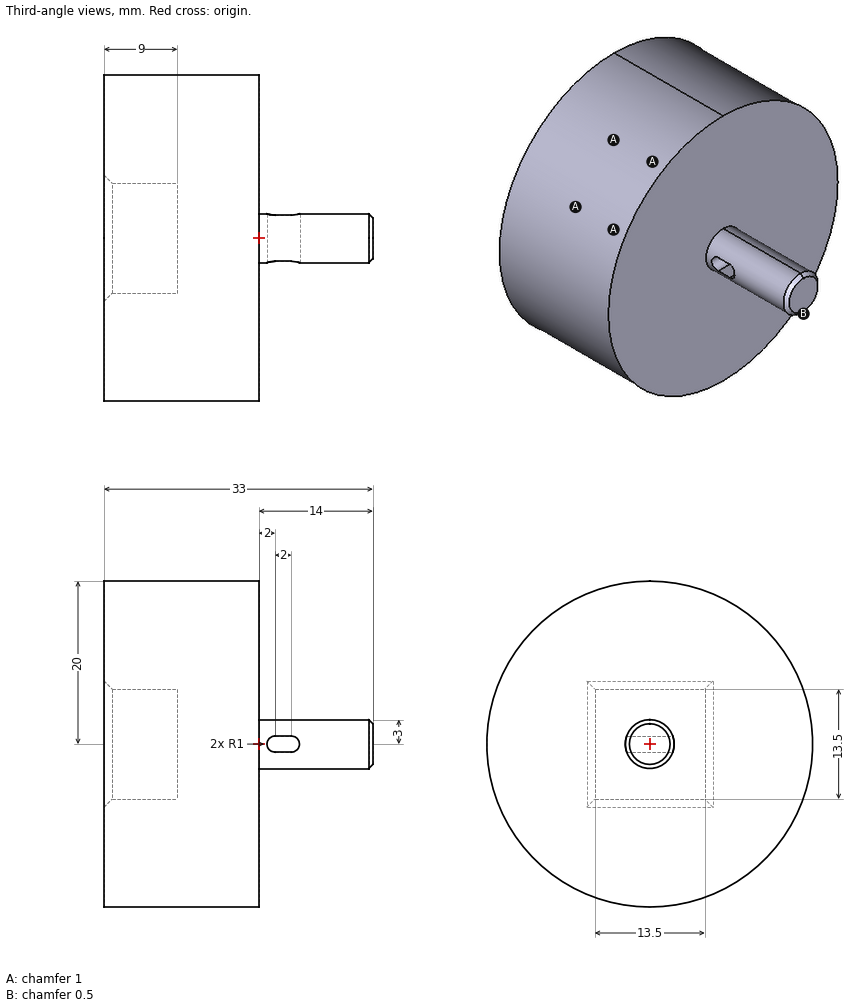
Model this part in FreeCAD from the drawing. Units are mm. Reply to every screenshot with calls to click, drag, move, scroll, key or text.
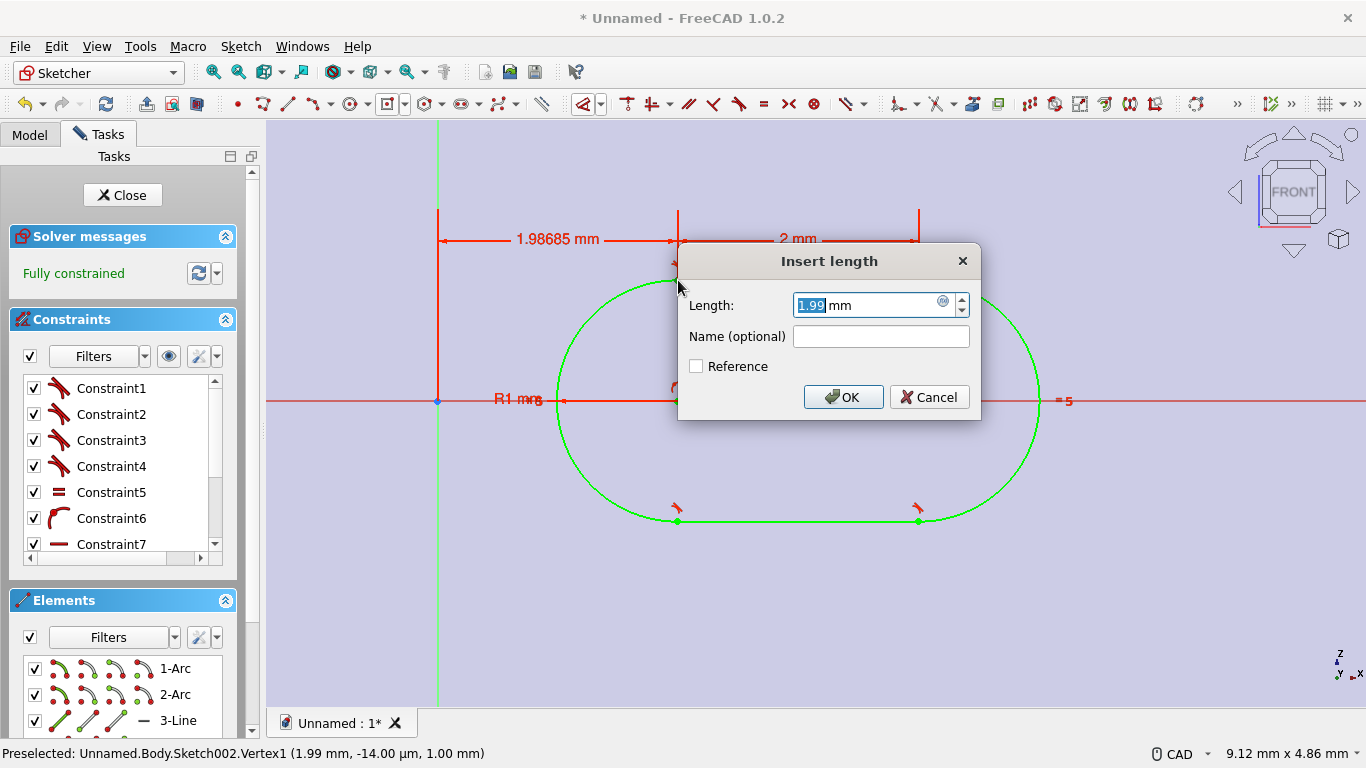
text(2)
key(Return)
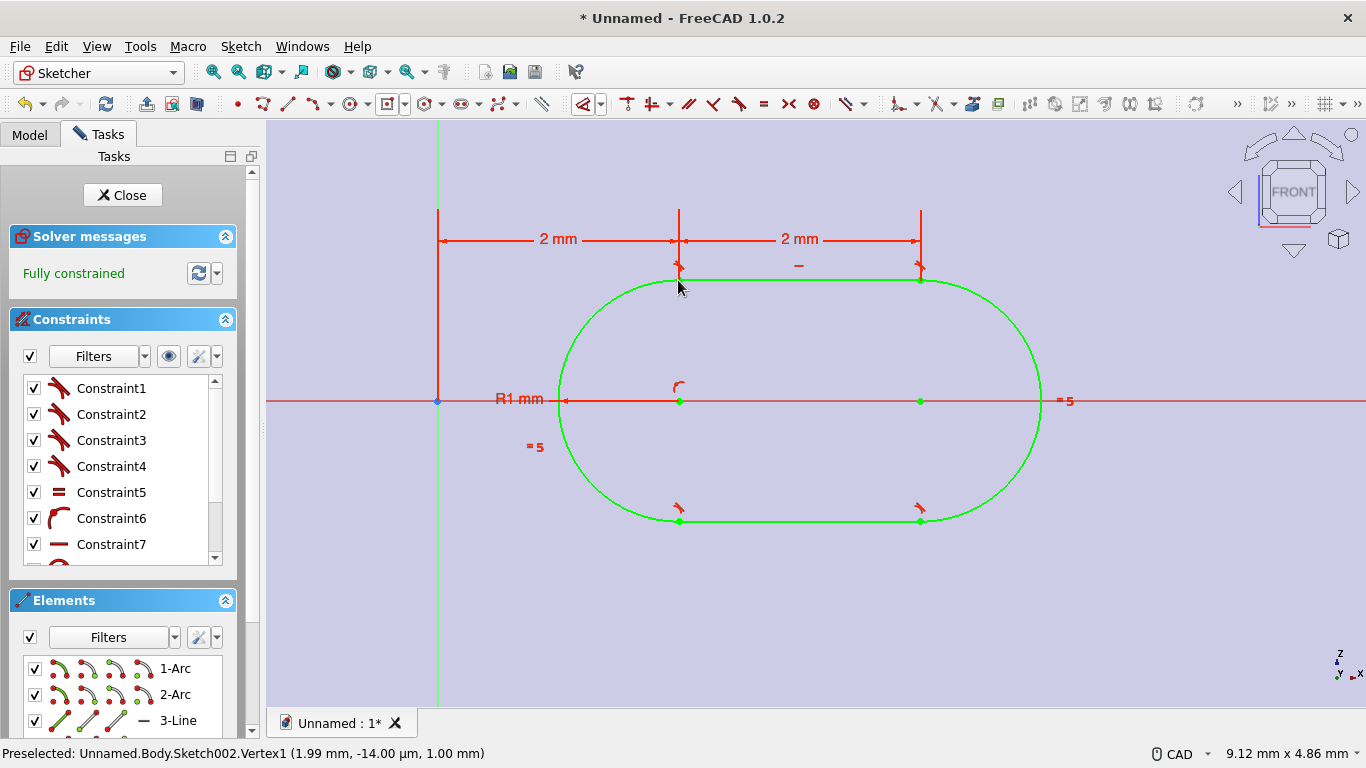
click(123, 195)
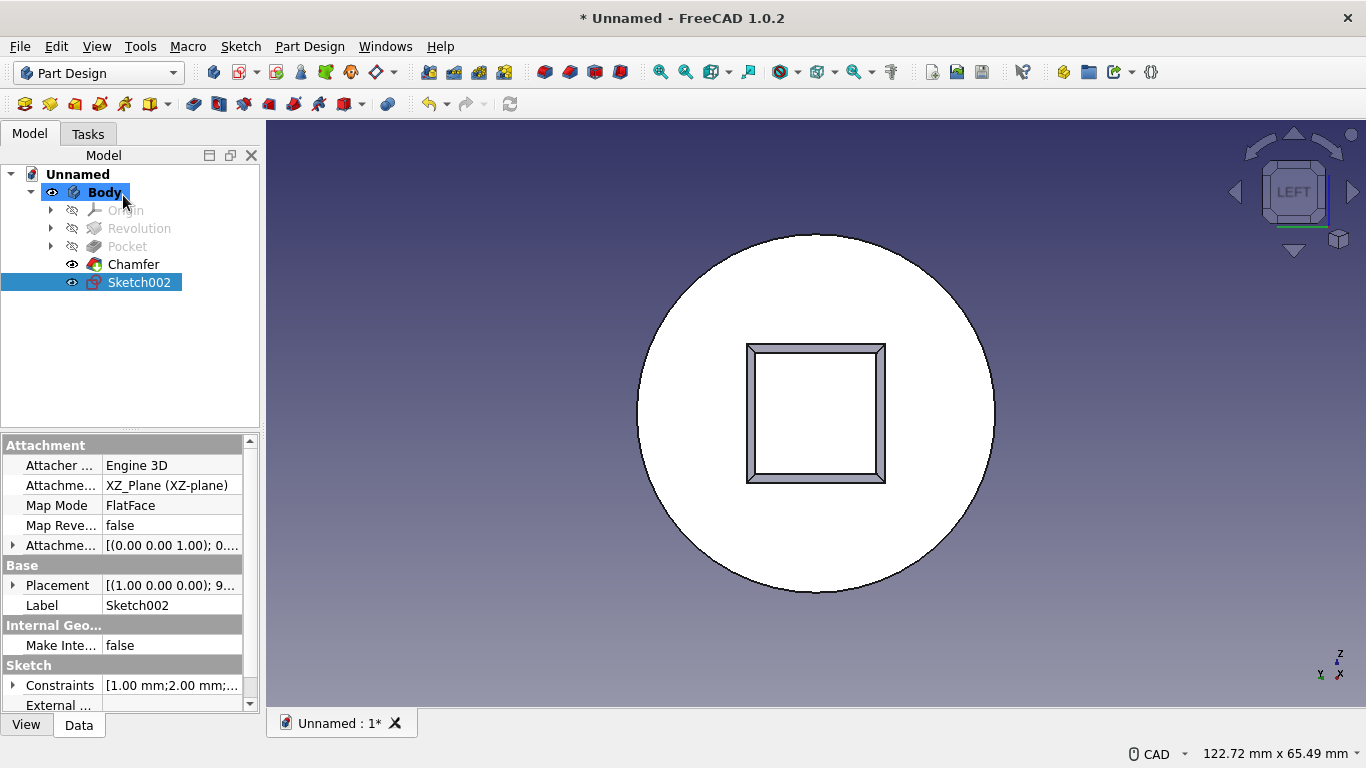
click(194, 104)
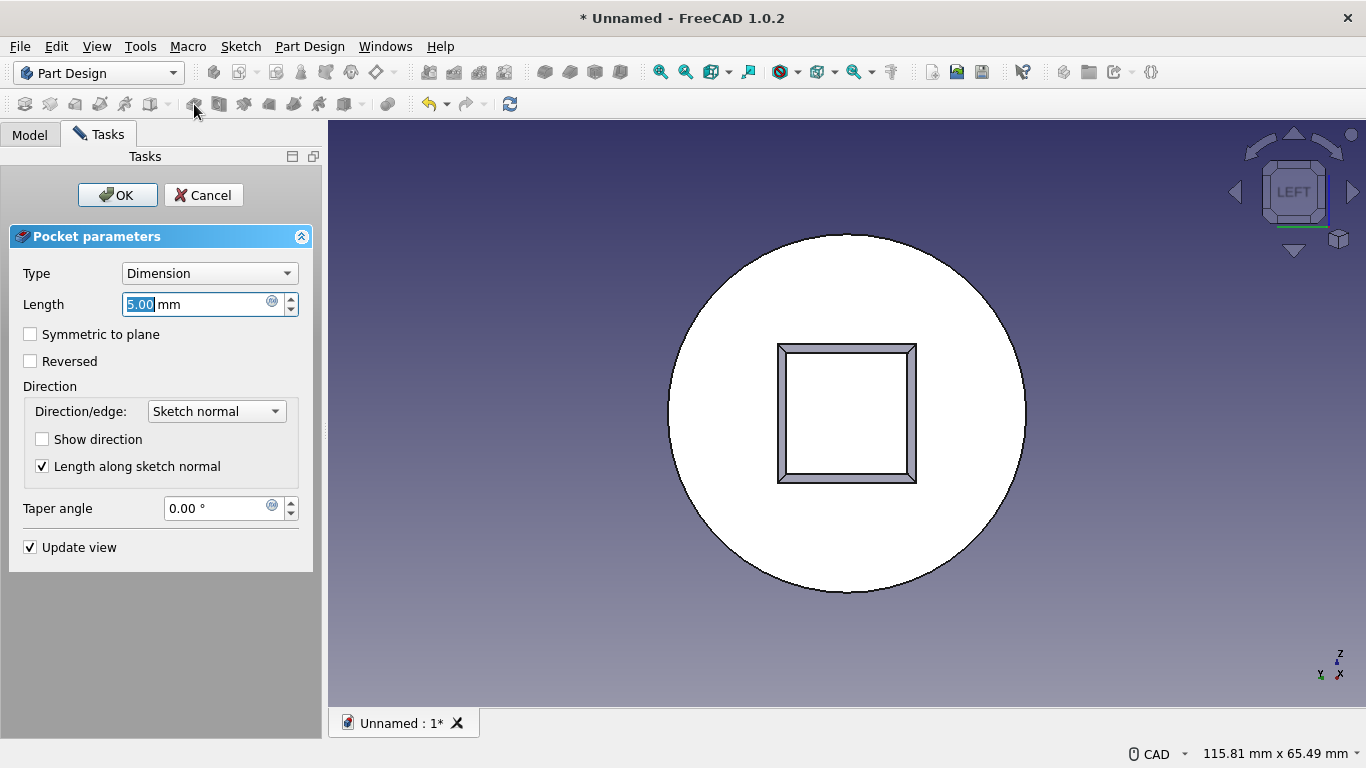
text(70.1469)
key(Tab)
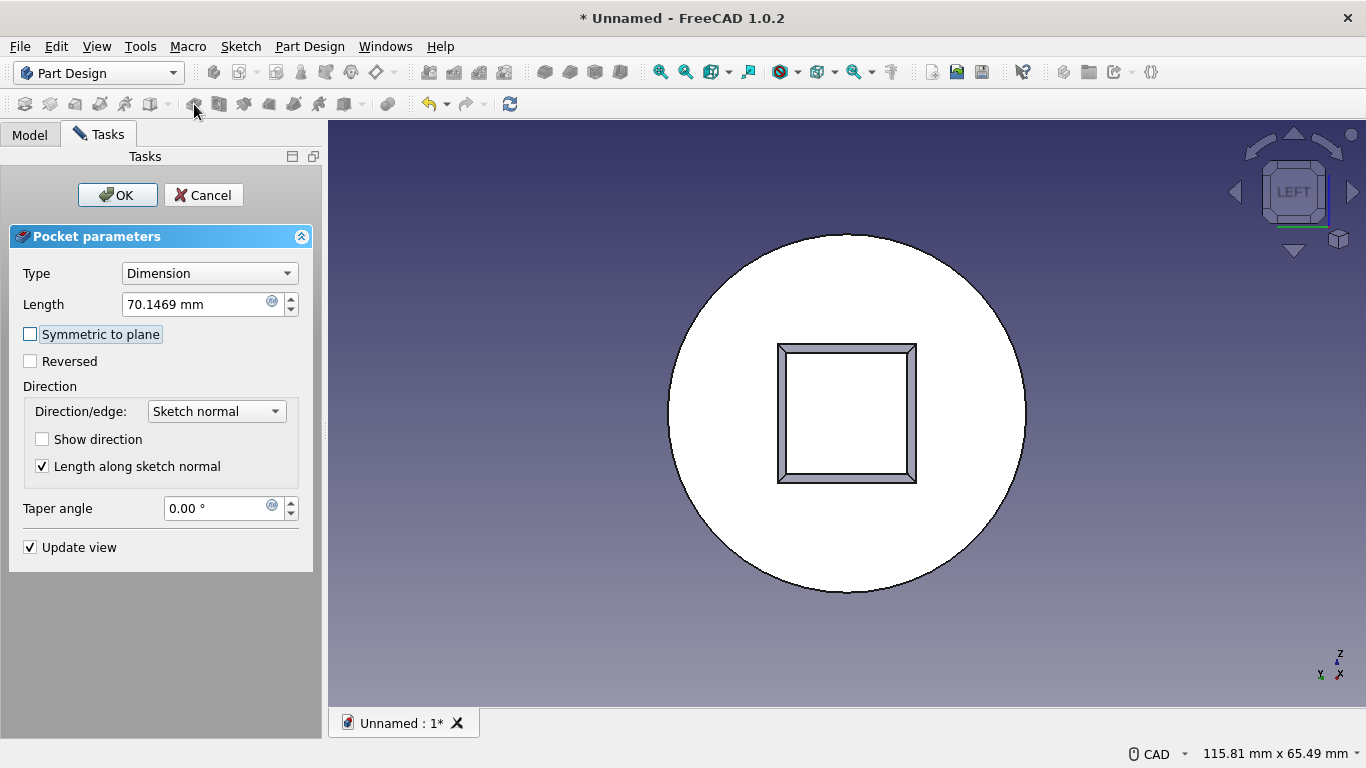
click(31, 334)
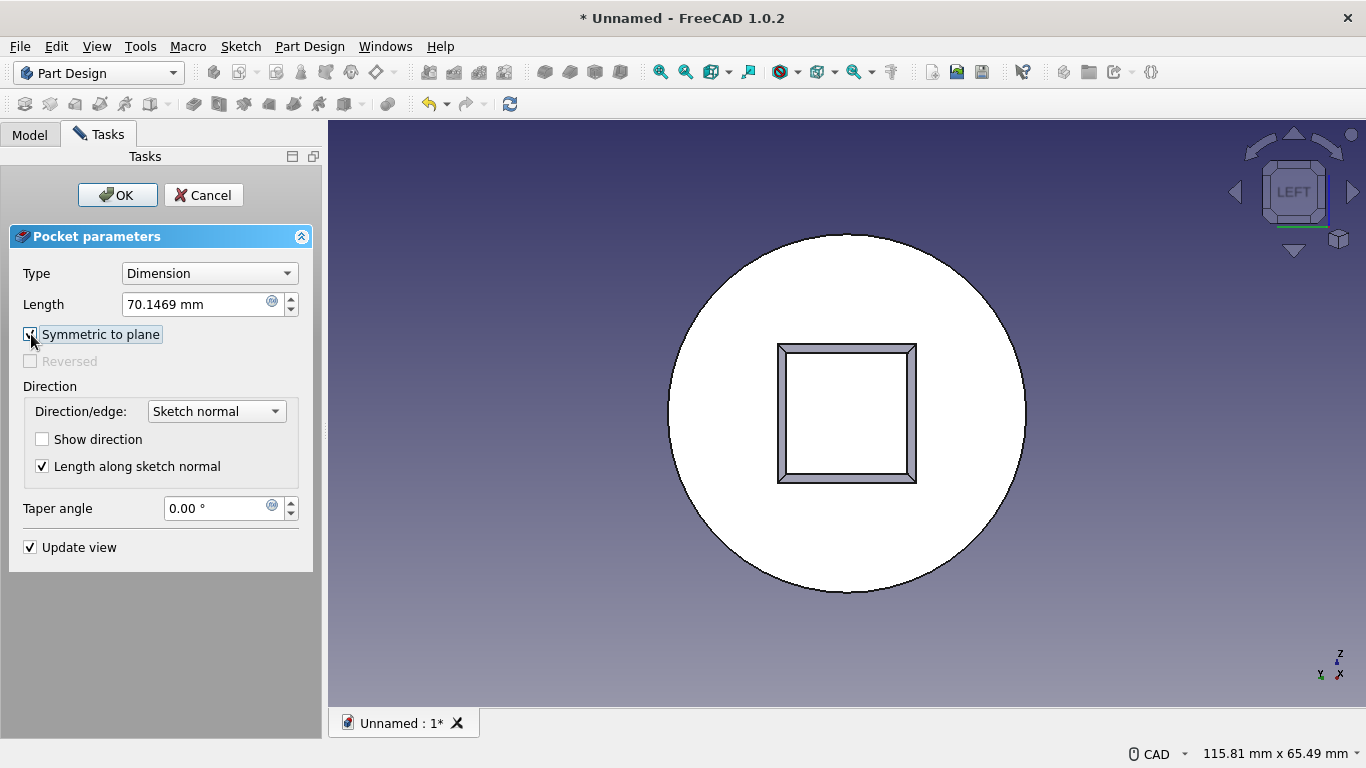
click(118, 195)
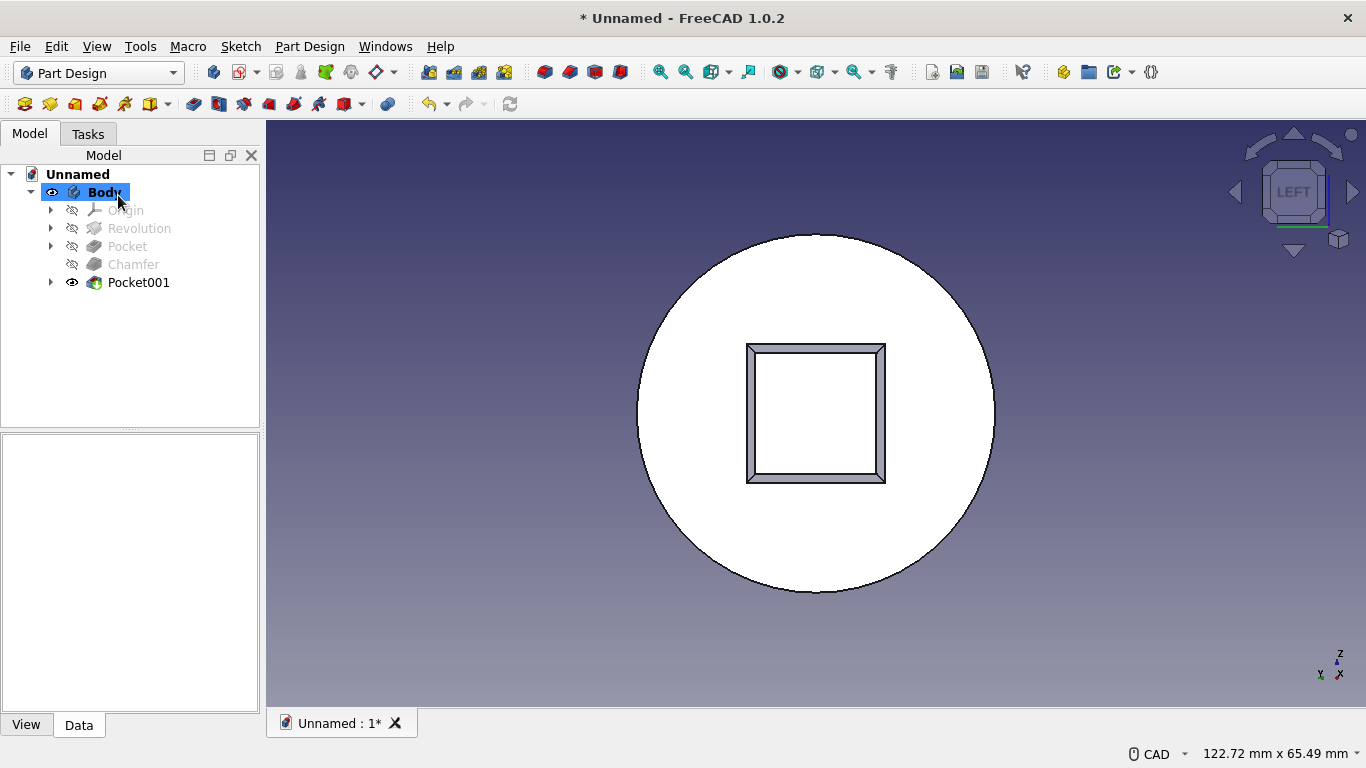
key(0)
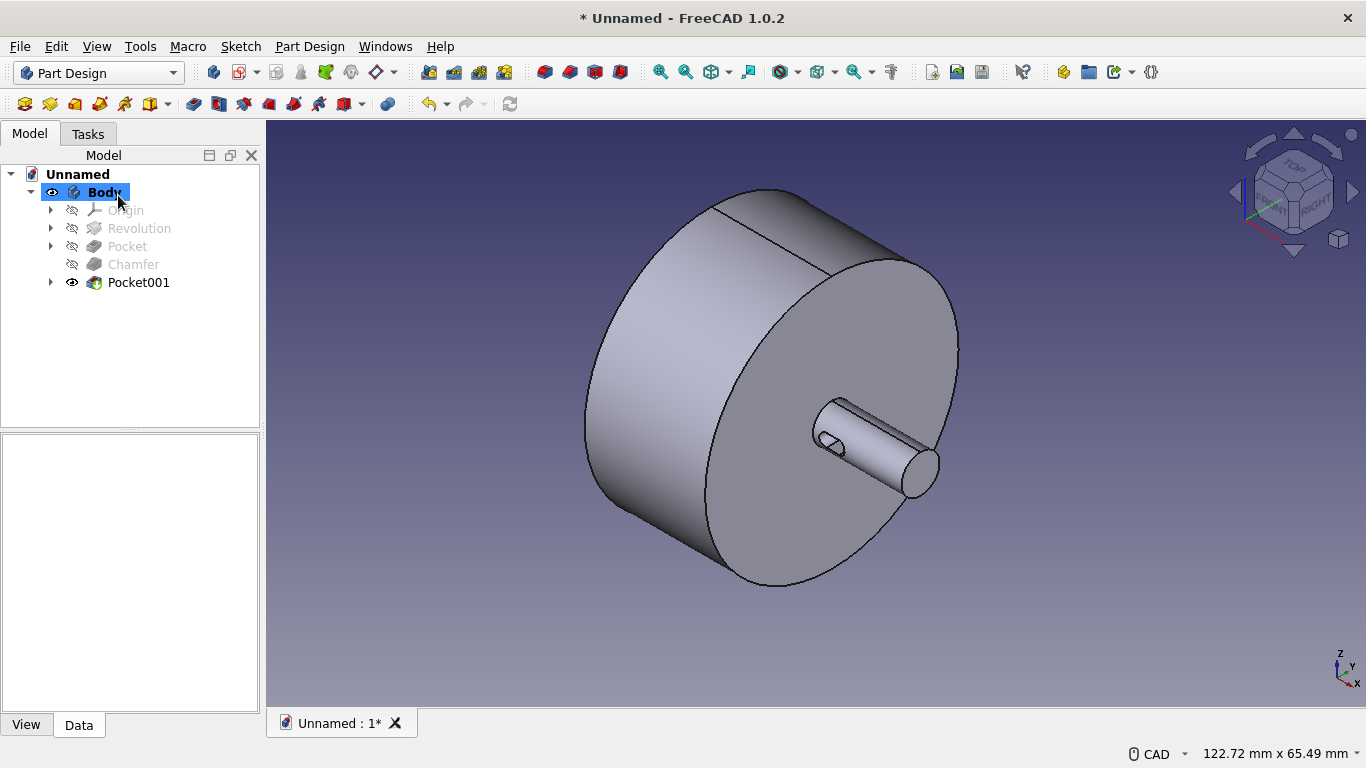
click(909, 497)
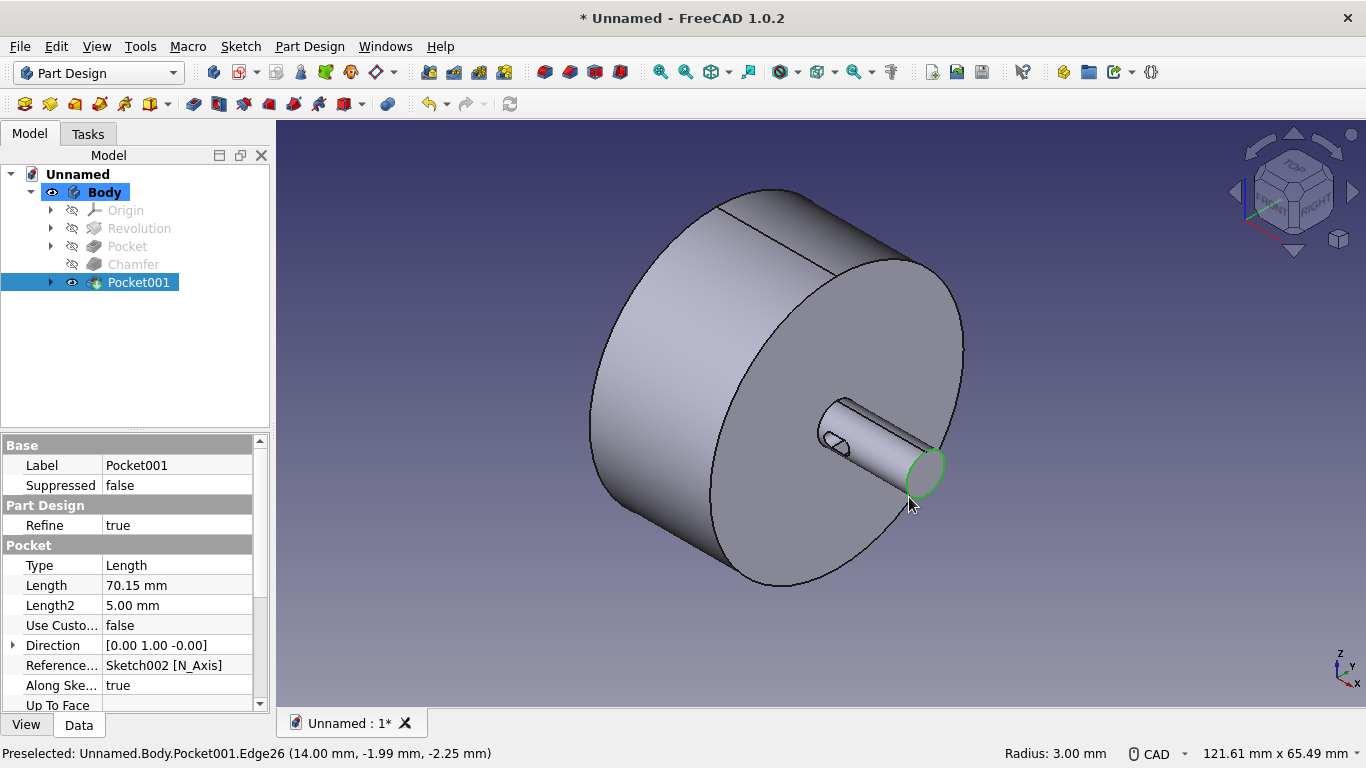
click(570, 72)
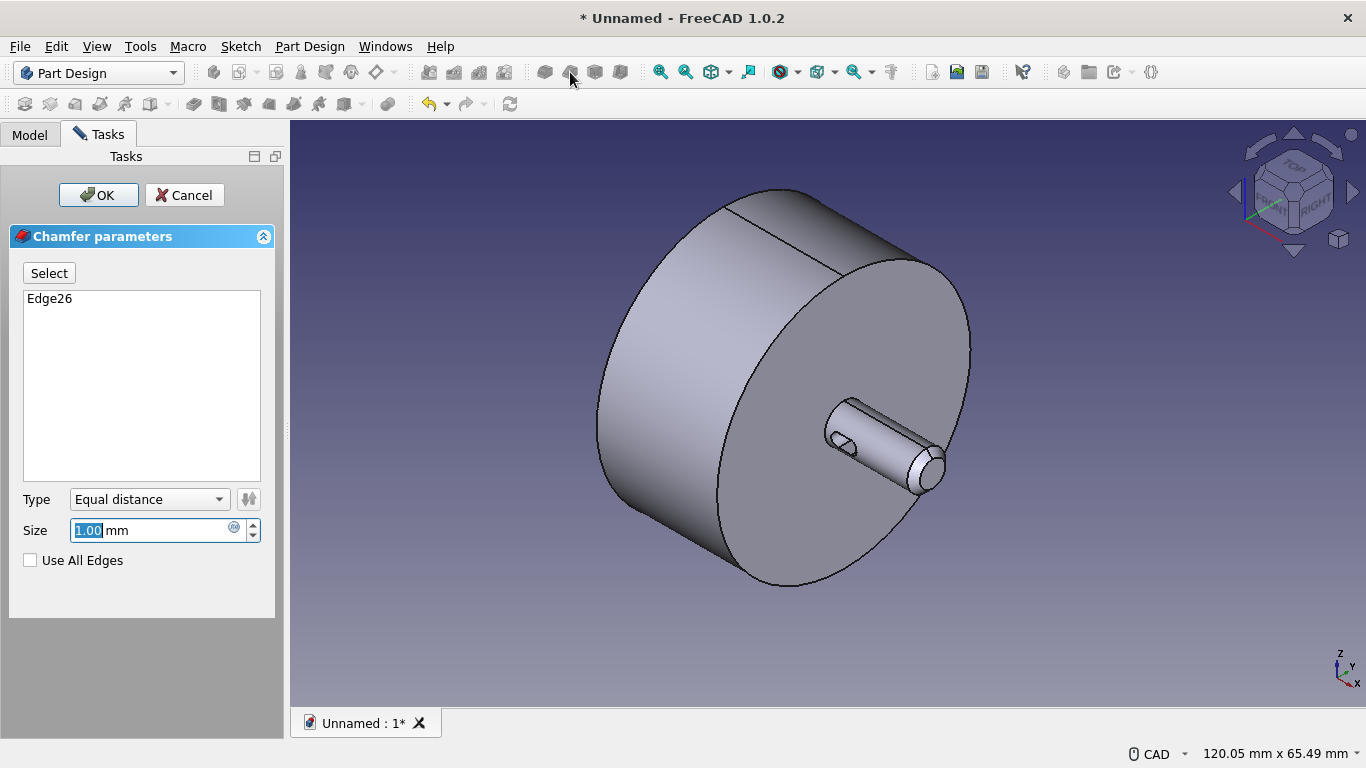
text(0.5)
key(Tab)